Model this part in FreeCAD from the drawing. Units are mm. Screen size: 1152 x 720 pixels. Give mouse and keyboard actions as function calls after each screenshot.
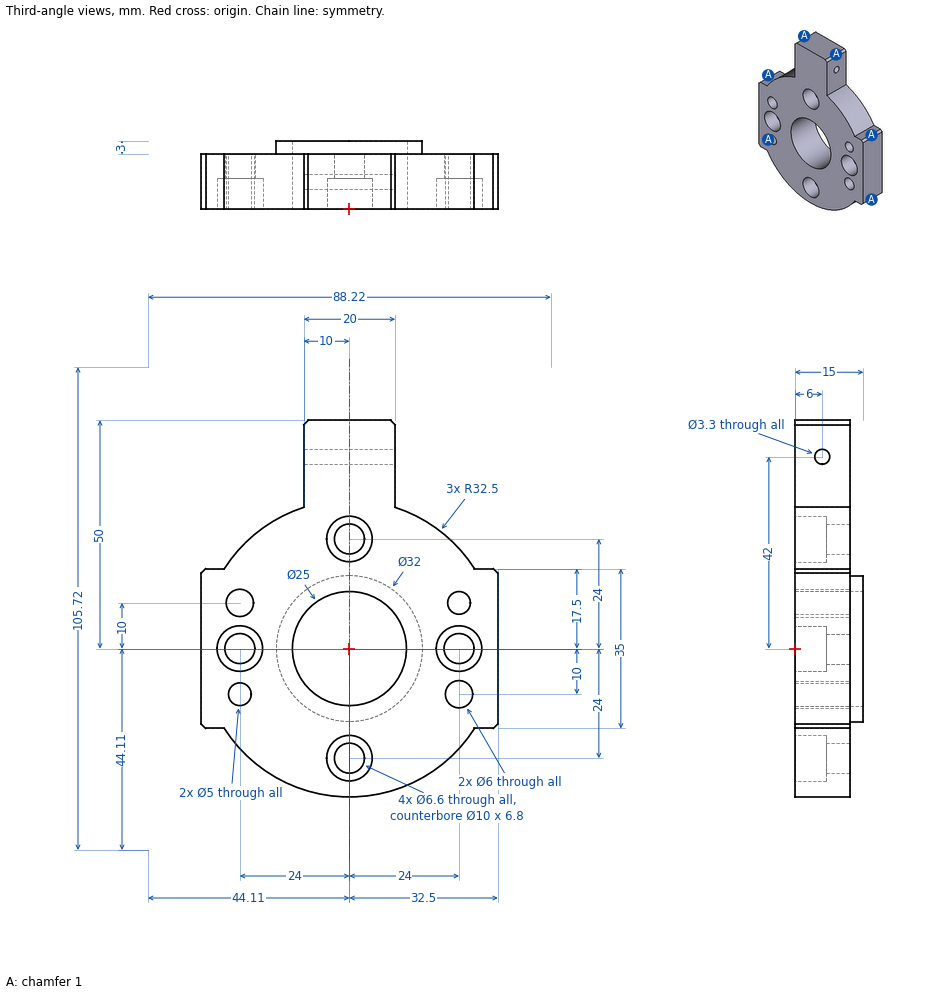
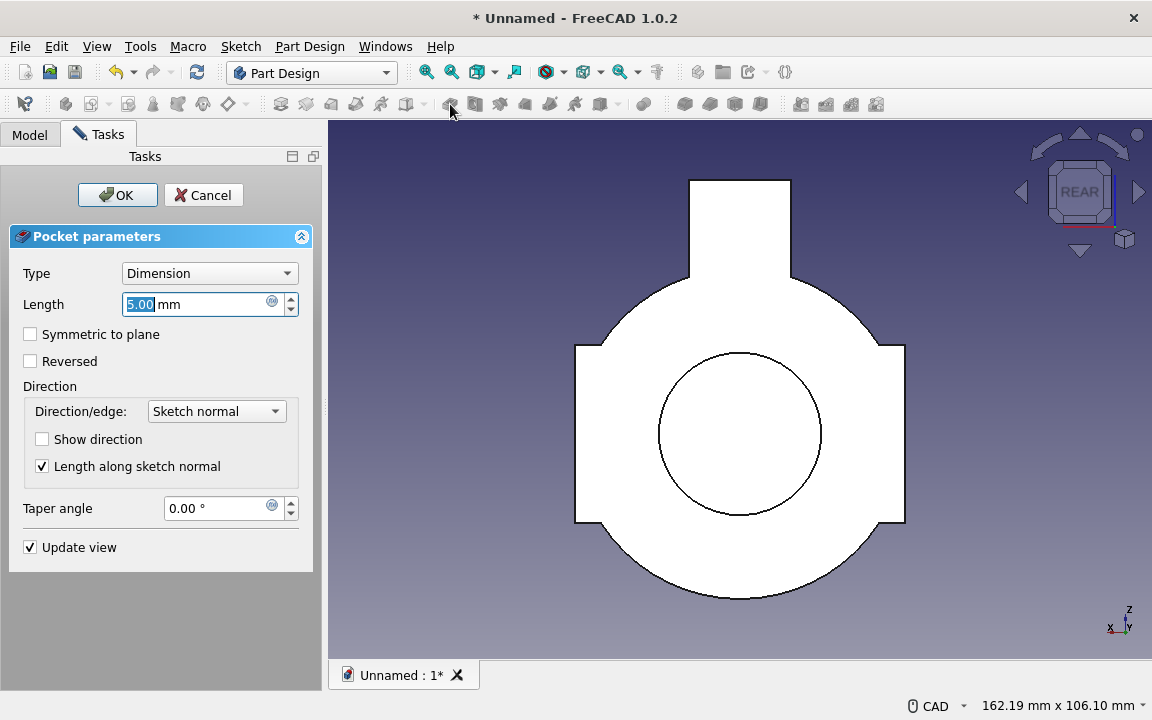
click(210, 274)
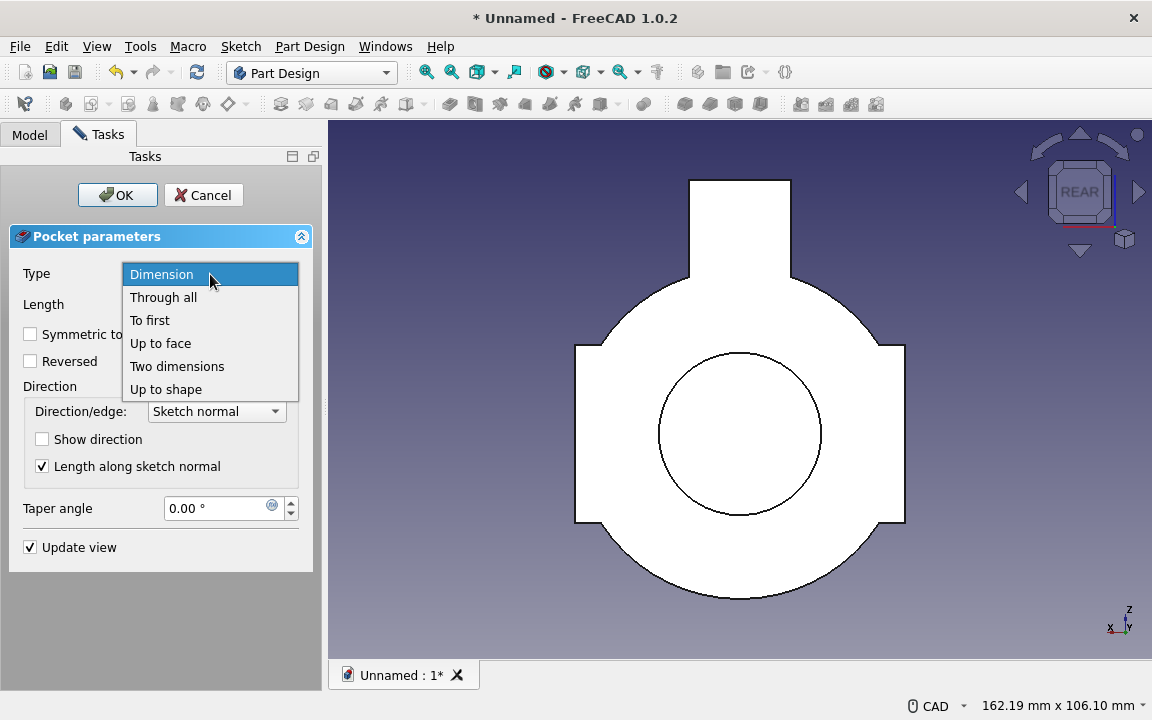
click(208, 298)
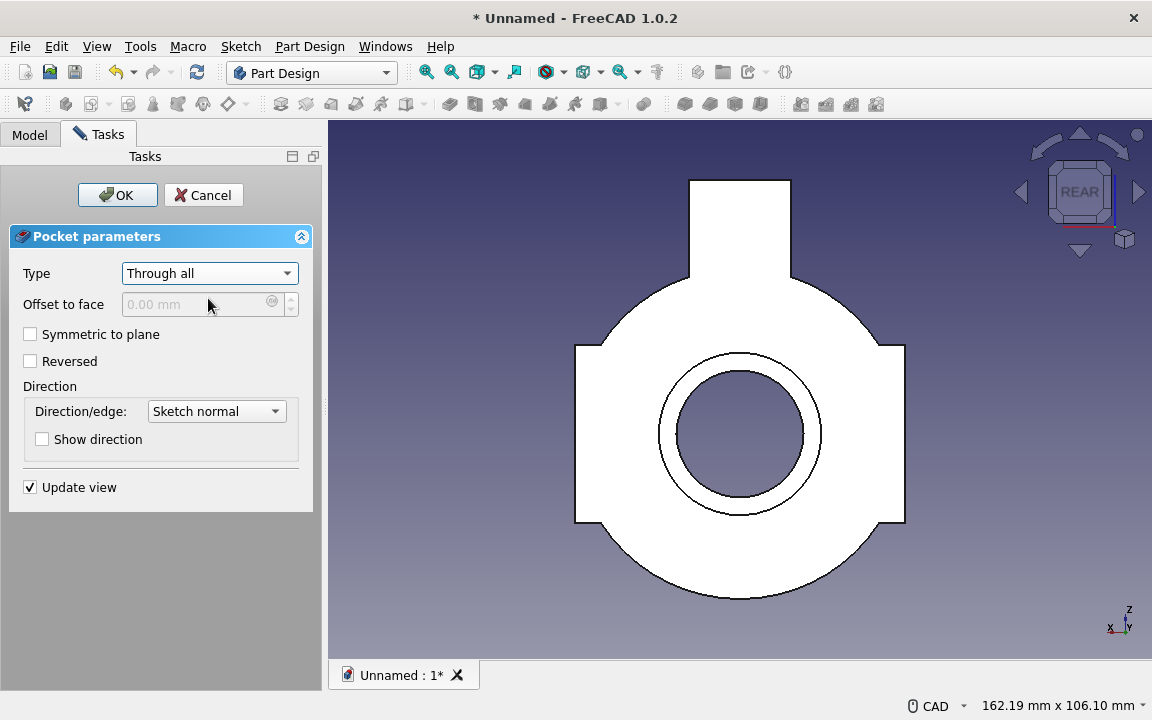
click(118, 195)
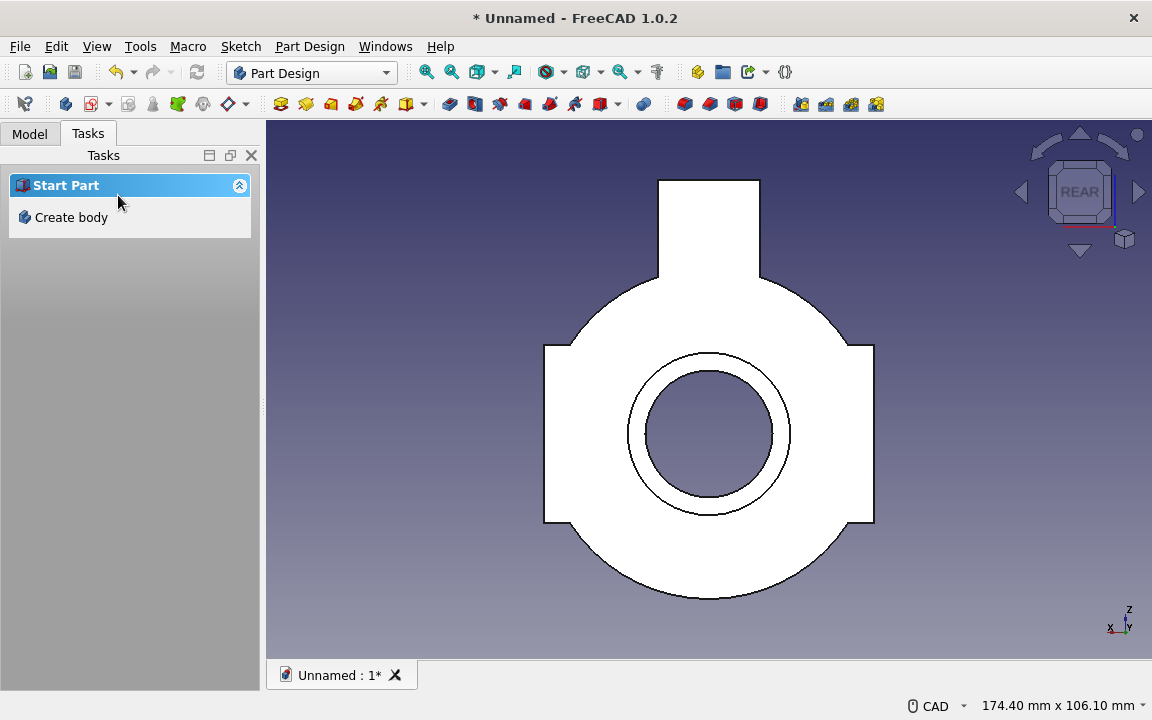
key(0)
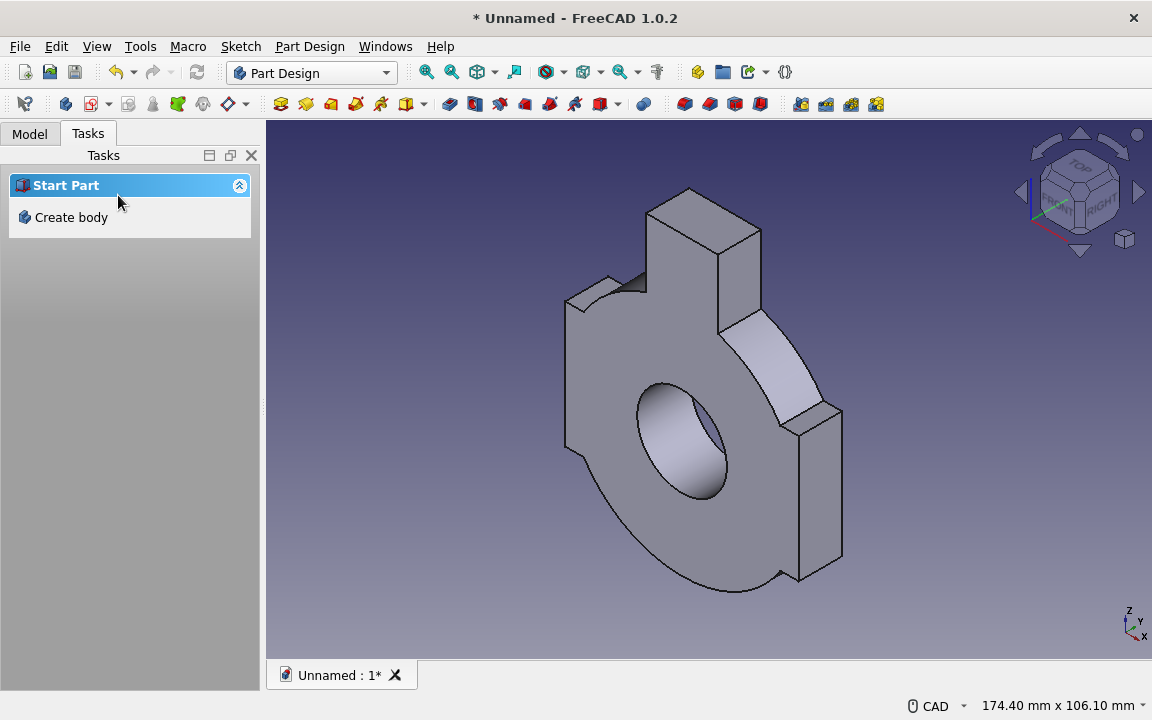
click(682, 306)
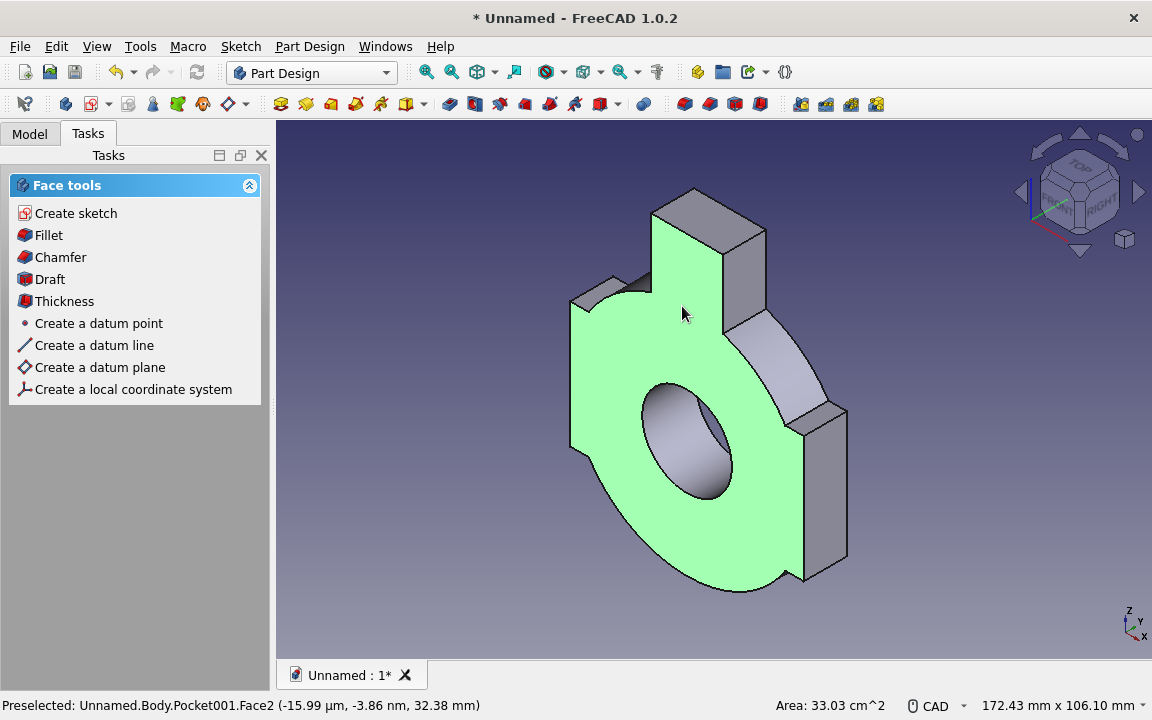
click(90, 104)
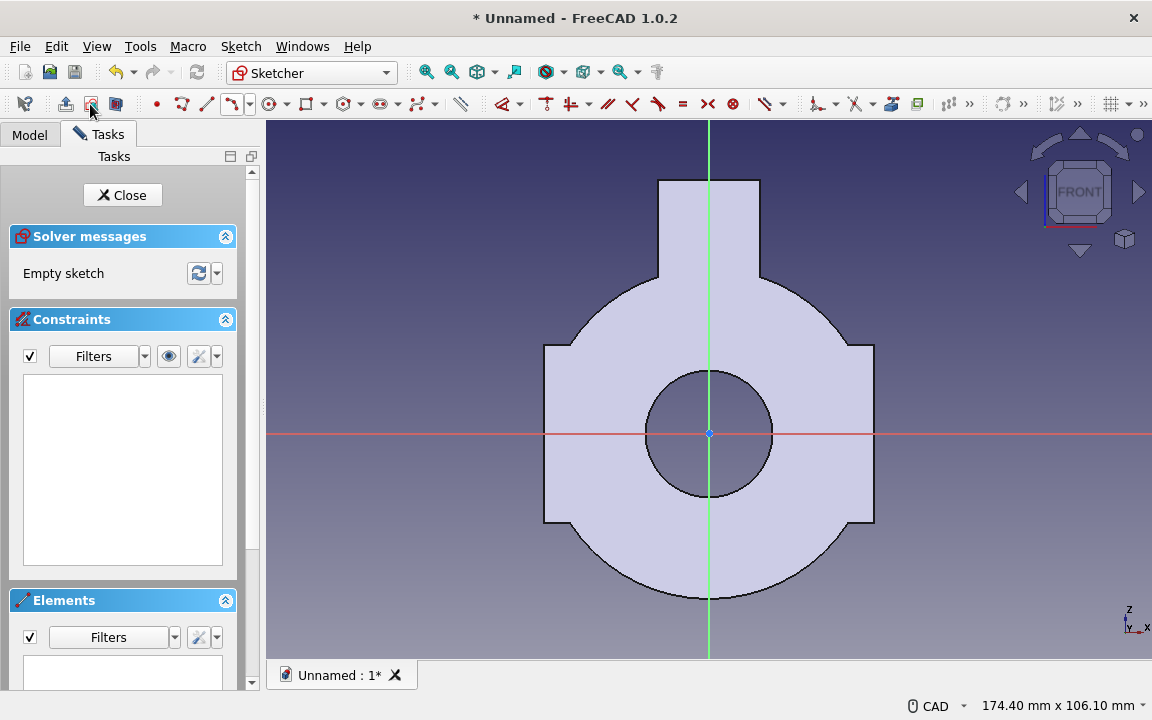
click(268, 104)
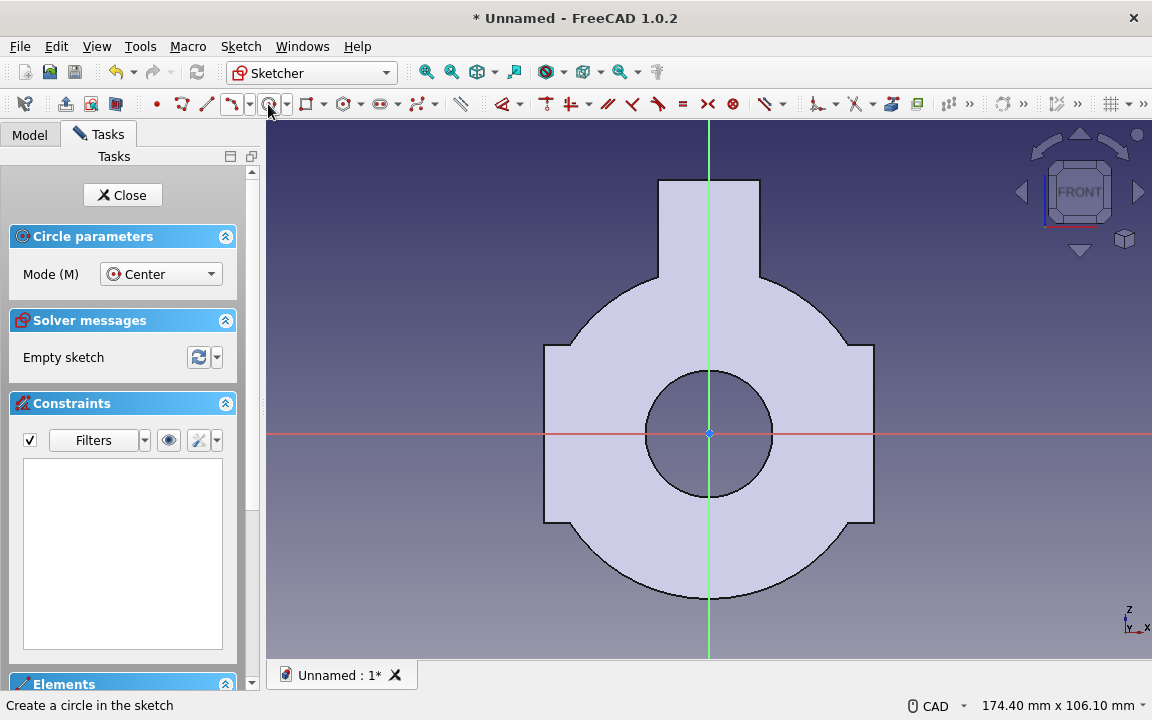
scroll(709, 556, up, 2)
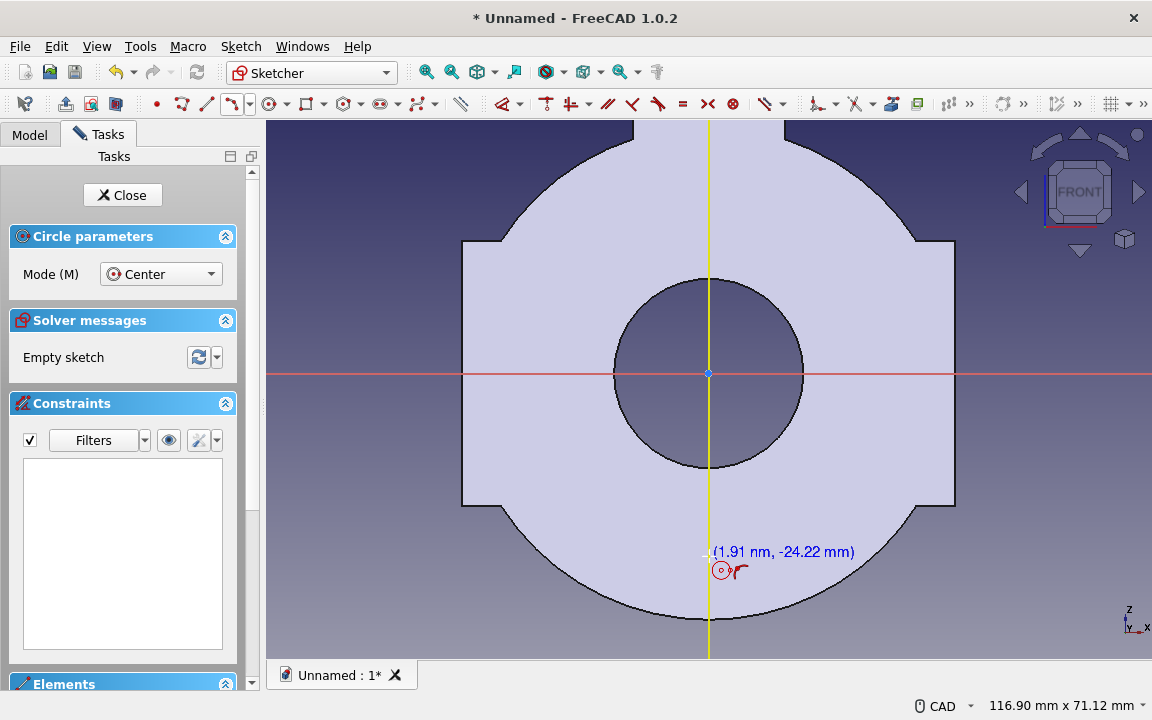
click(709, 555)
click(726, 538)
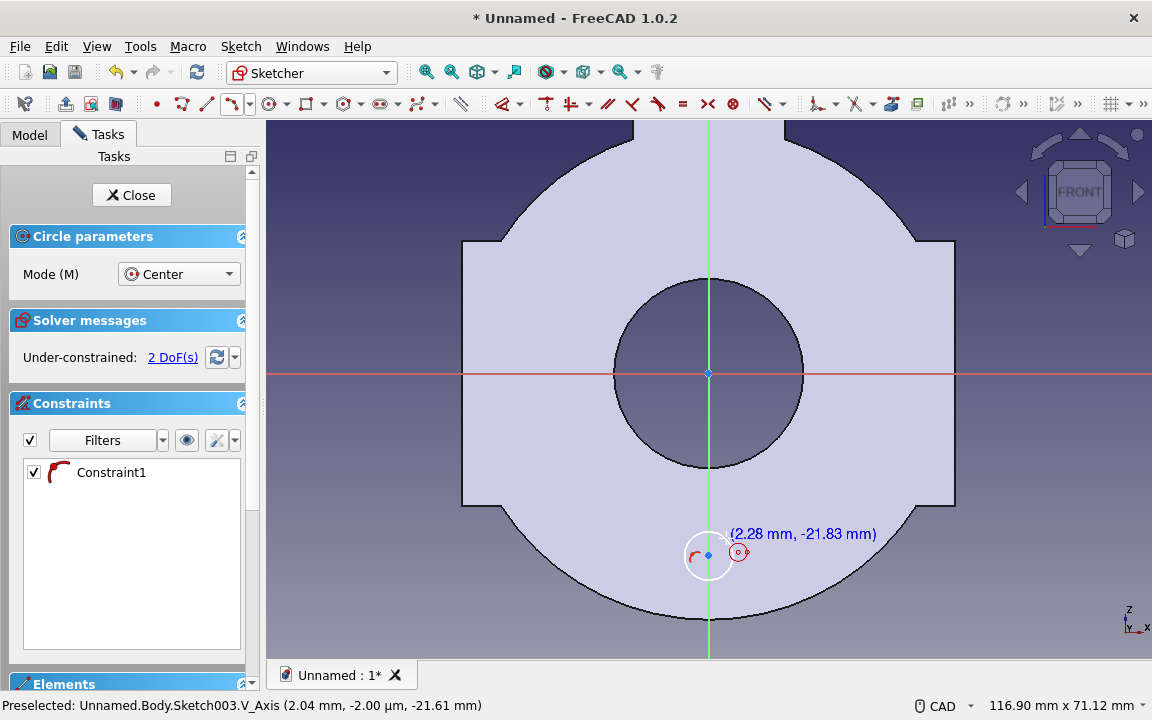
click(527, 374)
click(545, 356)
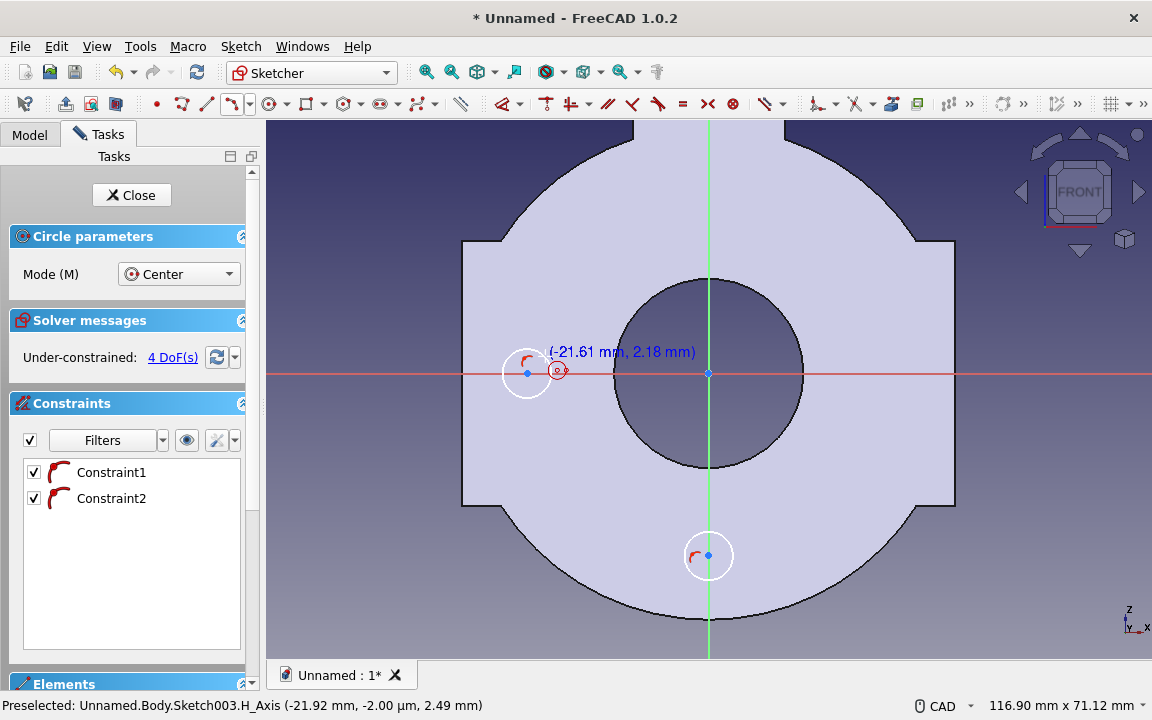
click(709, 192)
click(726, 174)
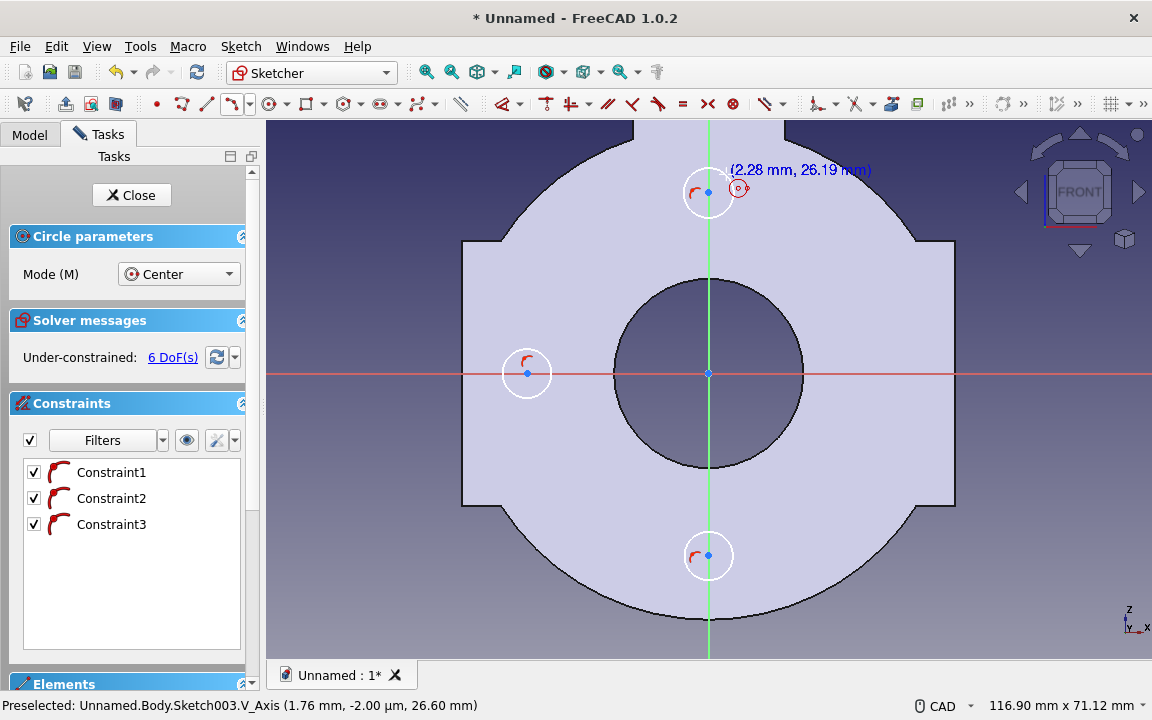
click(891, 374)
click(908, 356)
key(Escape)